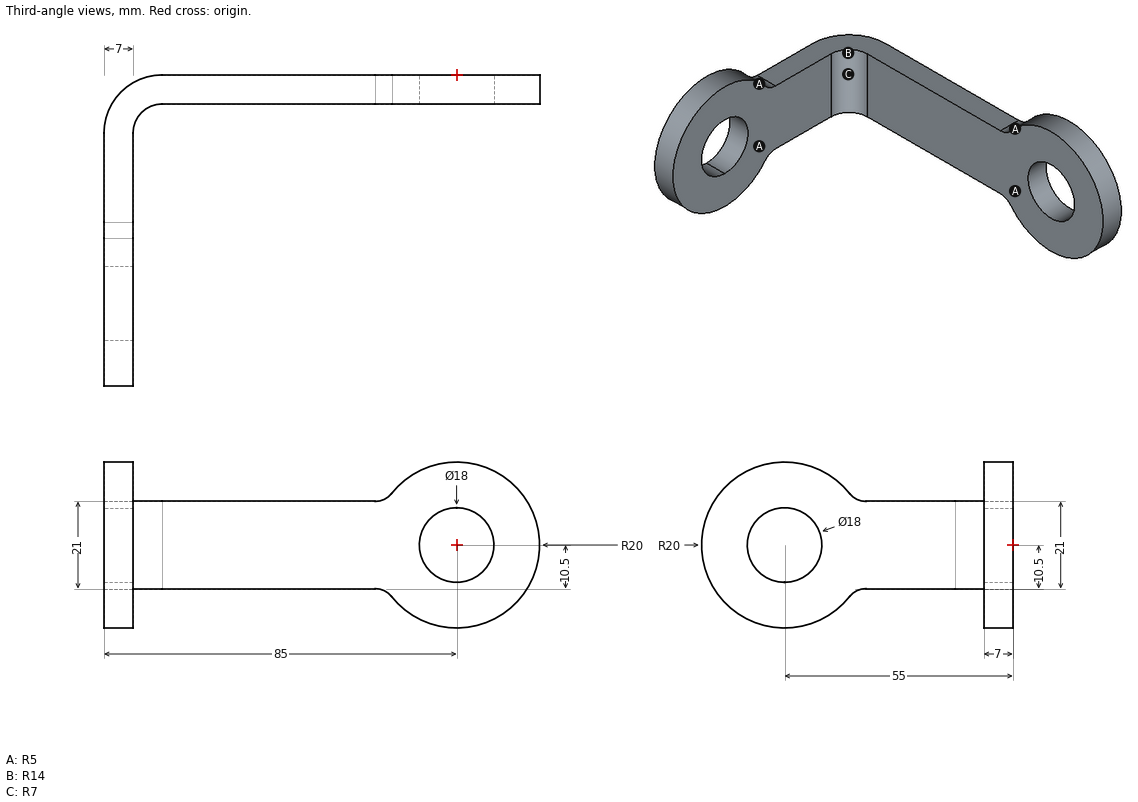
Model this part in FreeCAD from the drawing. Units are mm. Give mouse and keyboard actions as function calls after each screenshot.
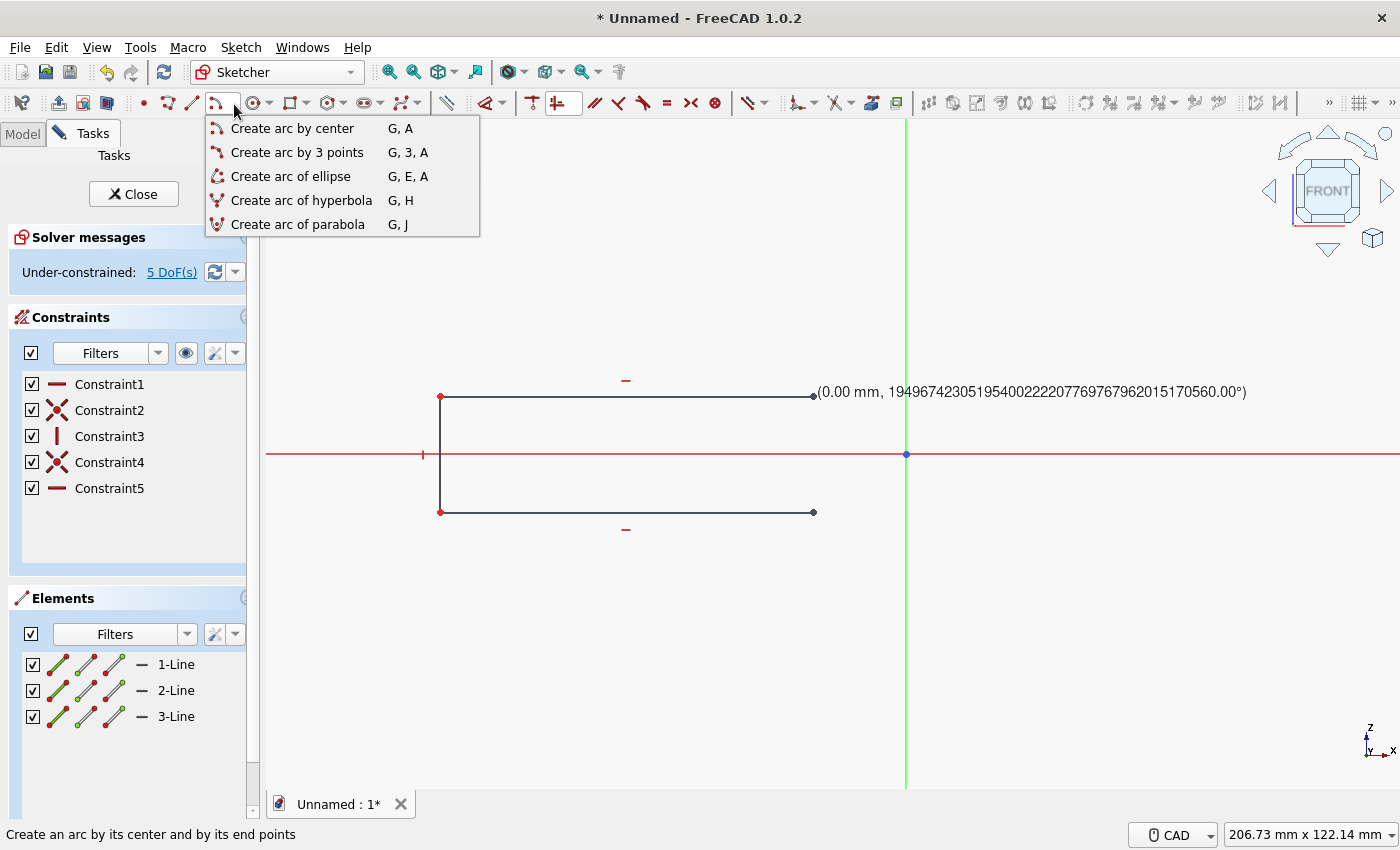
click(342, 152)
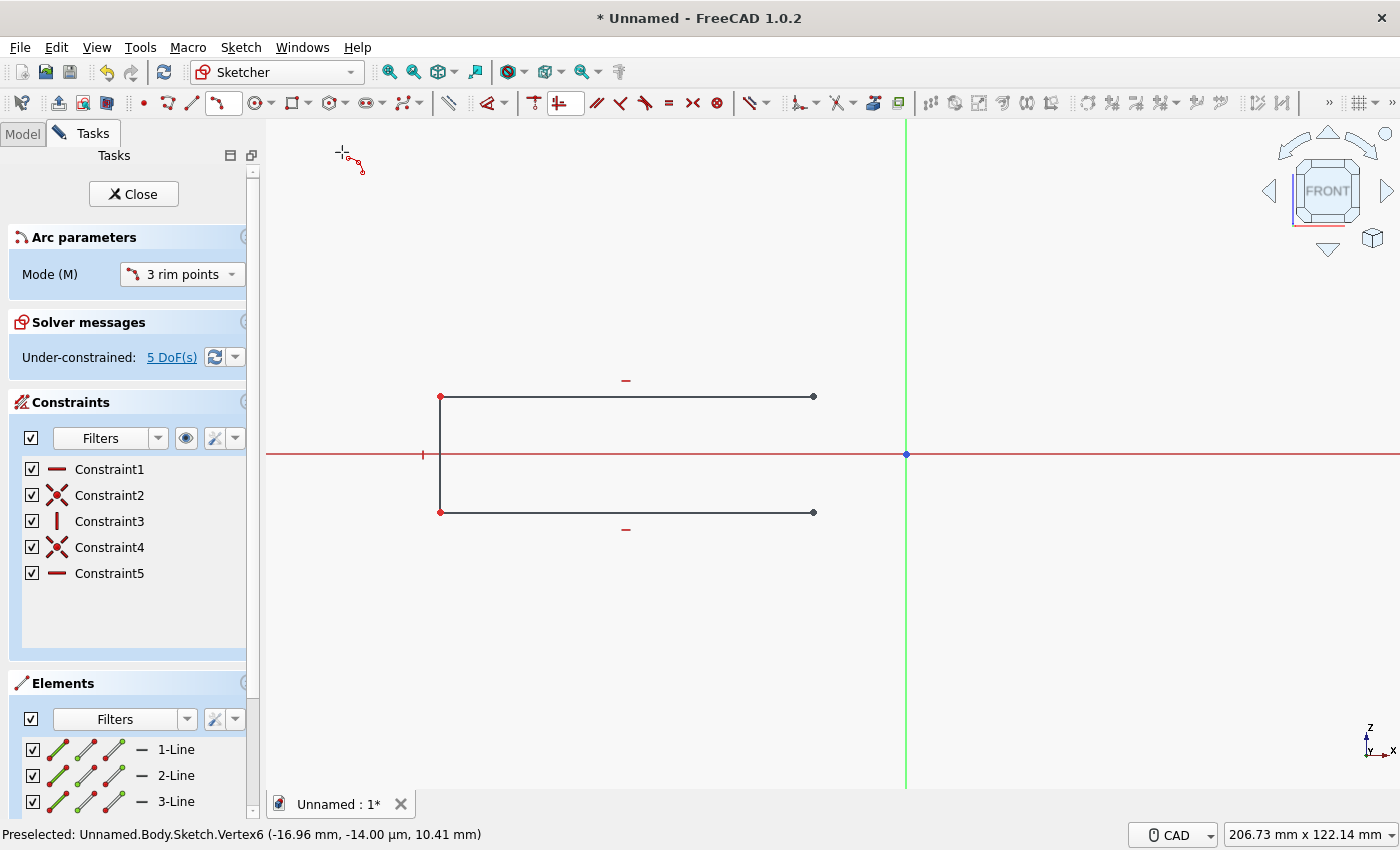
click(813, 397)
click(813, 513)
click(1001, 508)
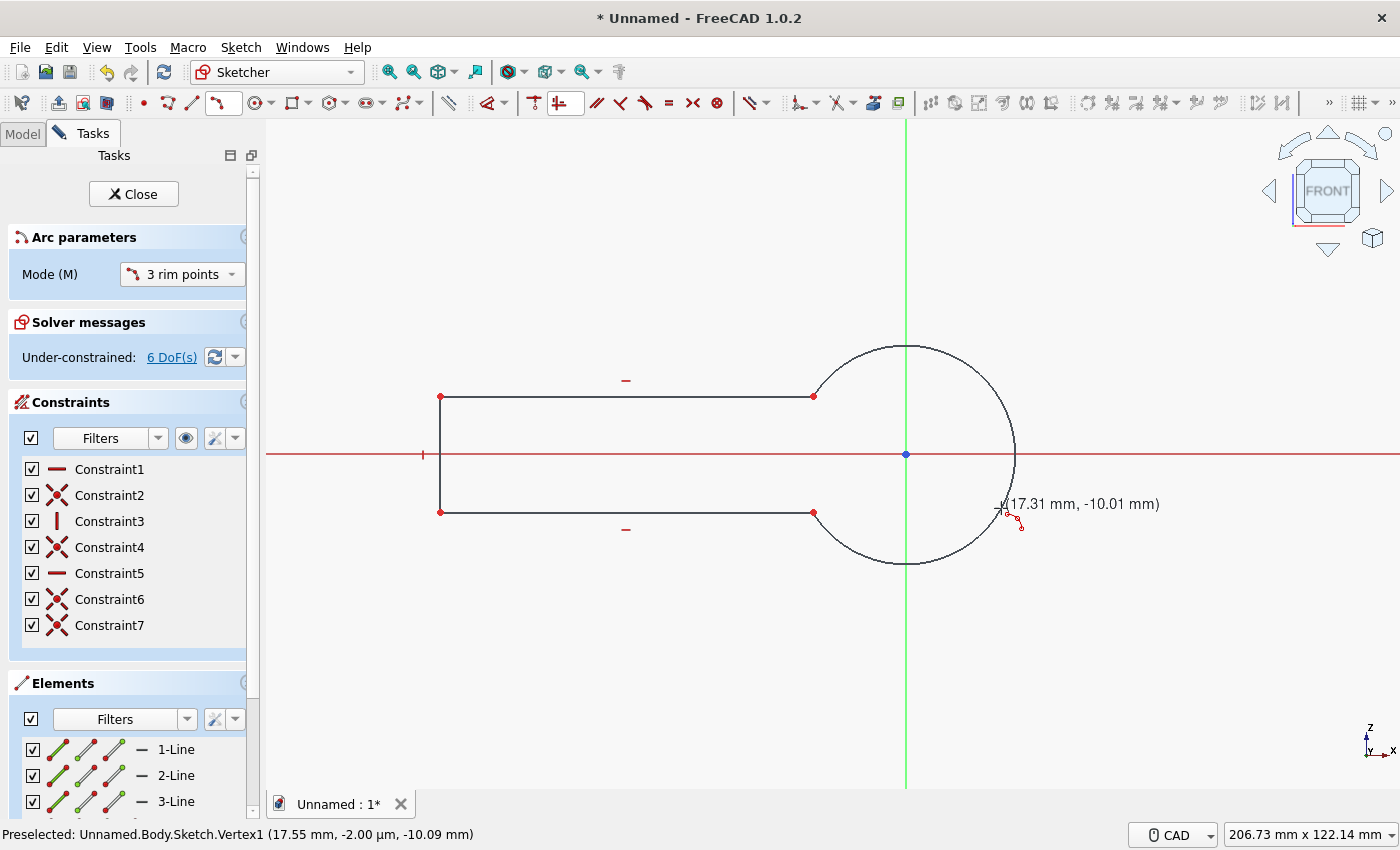
click(256, 104)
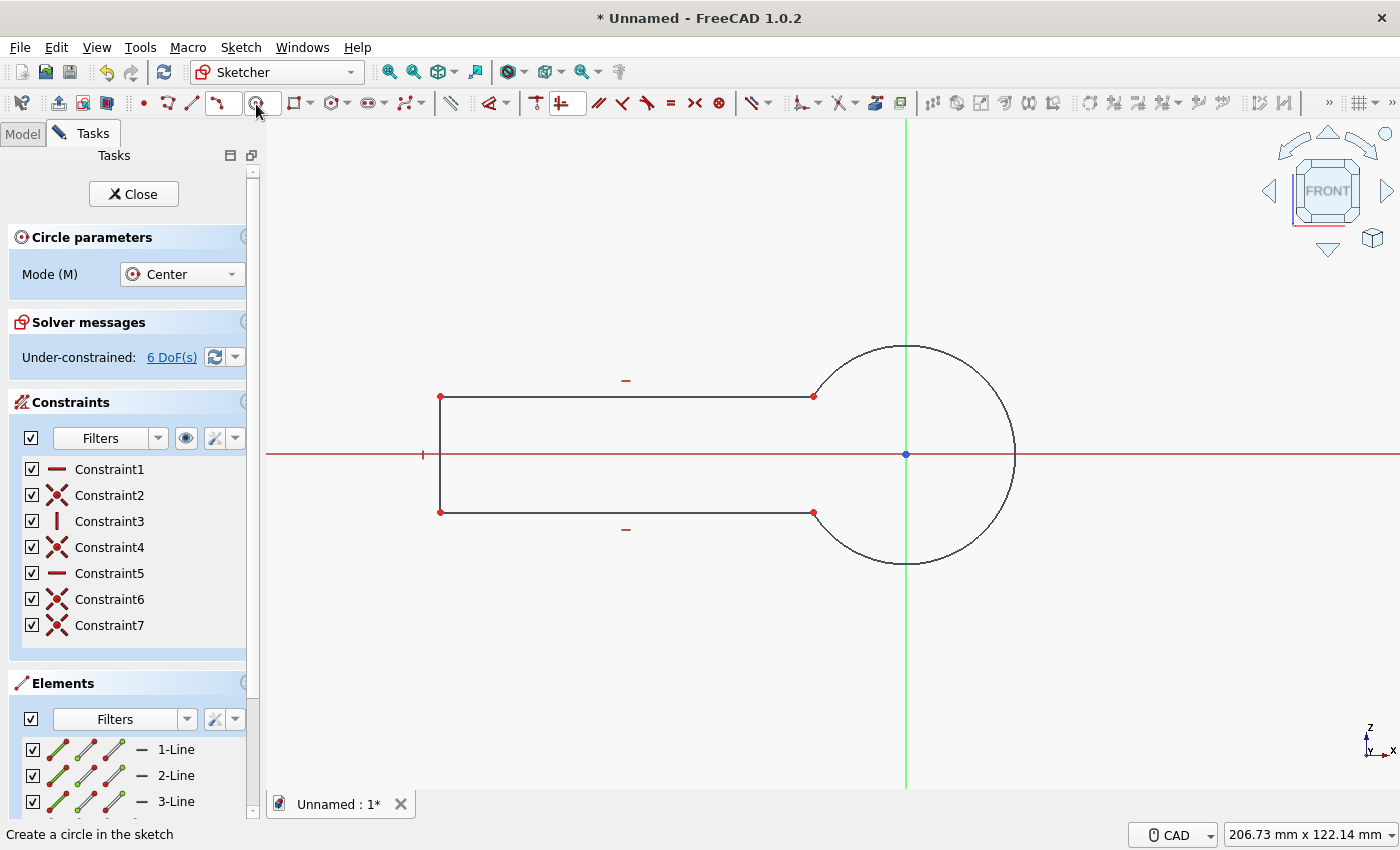
click(906, 454)
move(941, 419)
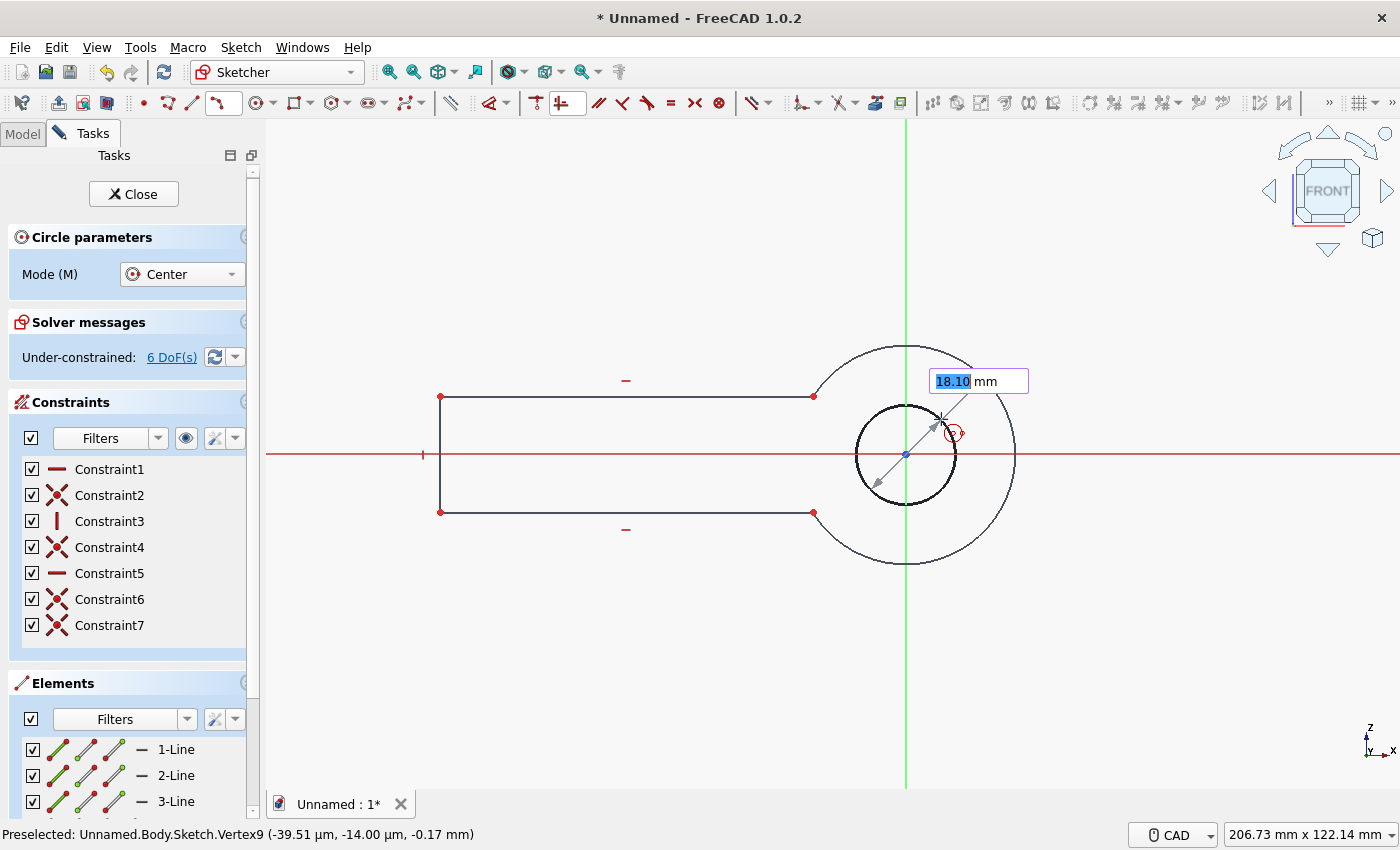
text(18)
key(Return)
key(Escape)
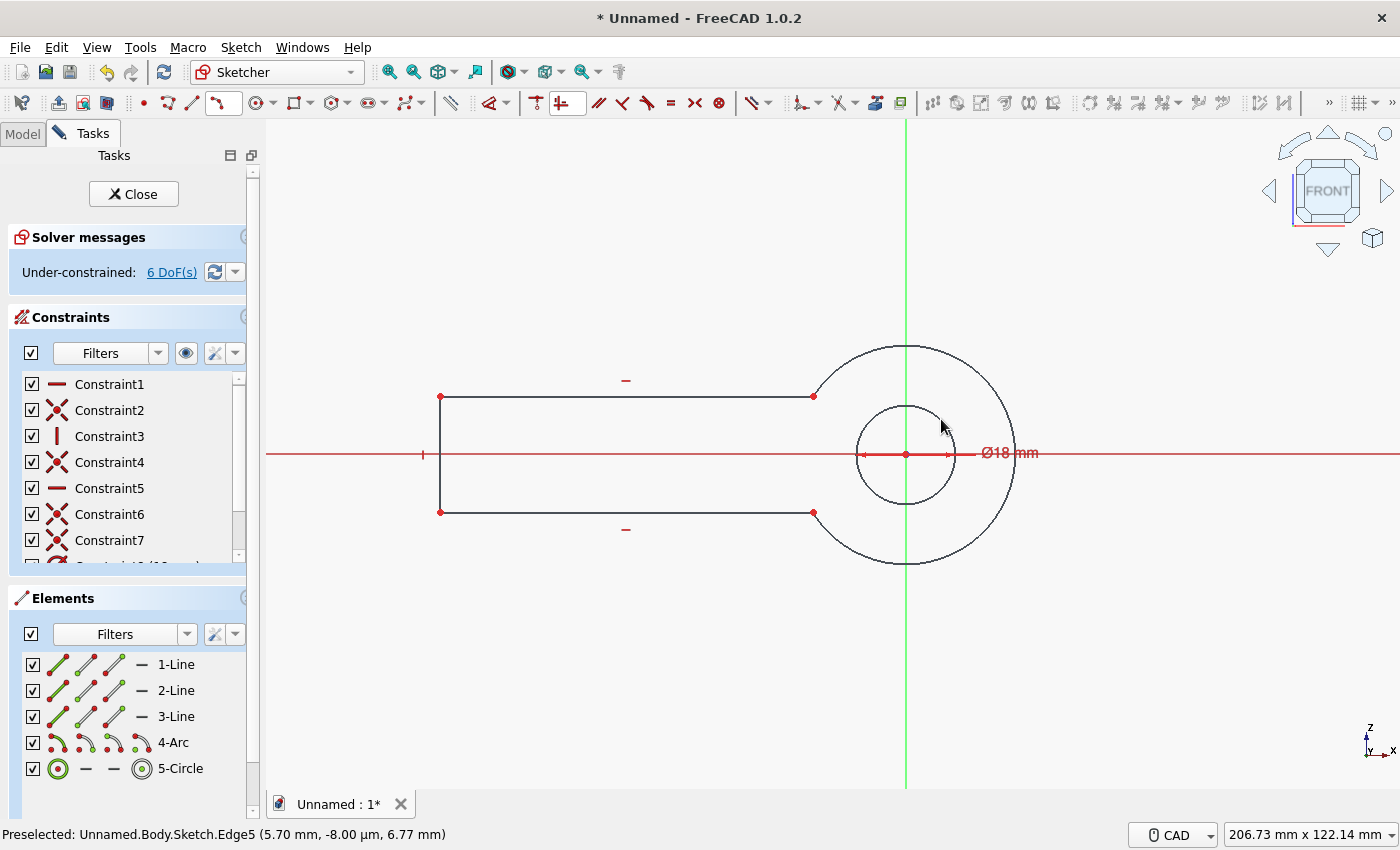
drag(896, 444, 916, 465)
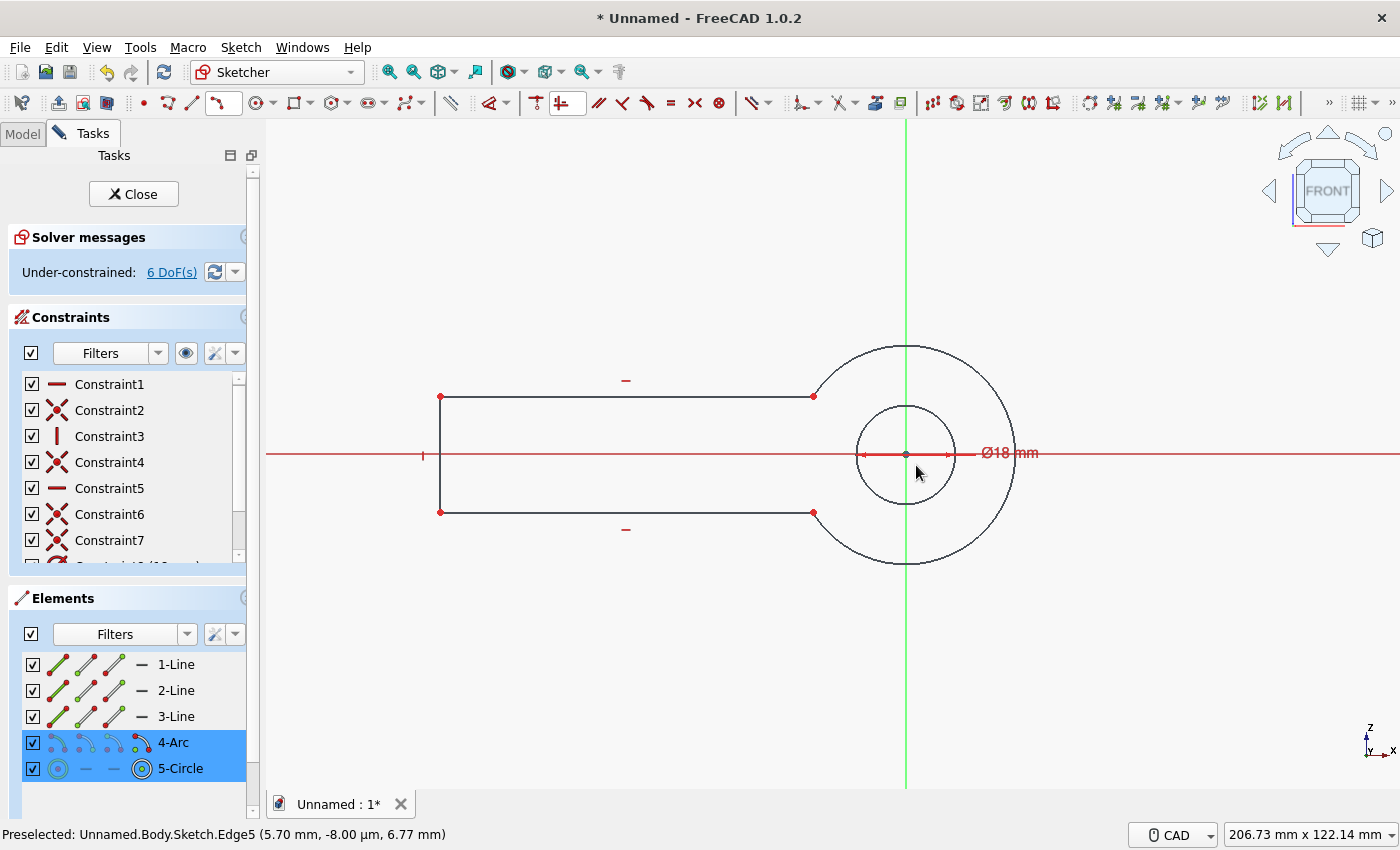
click(536, 104)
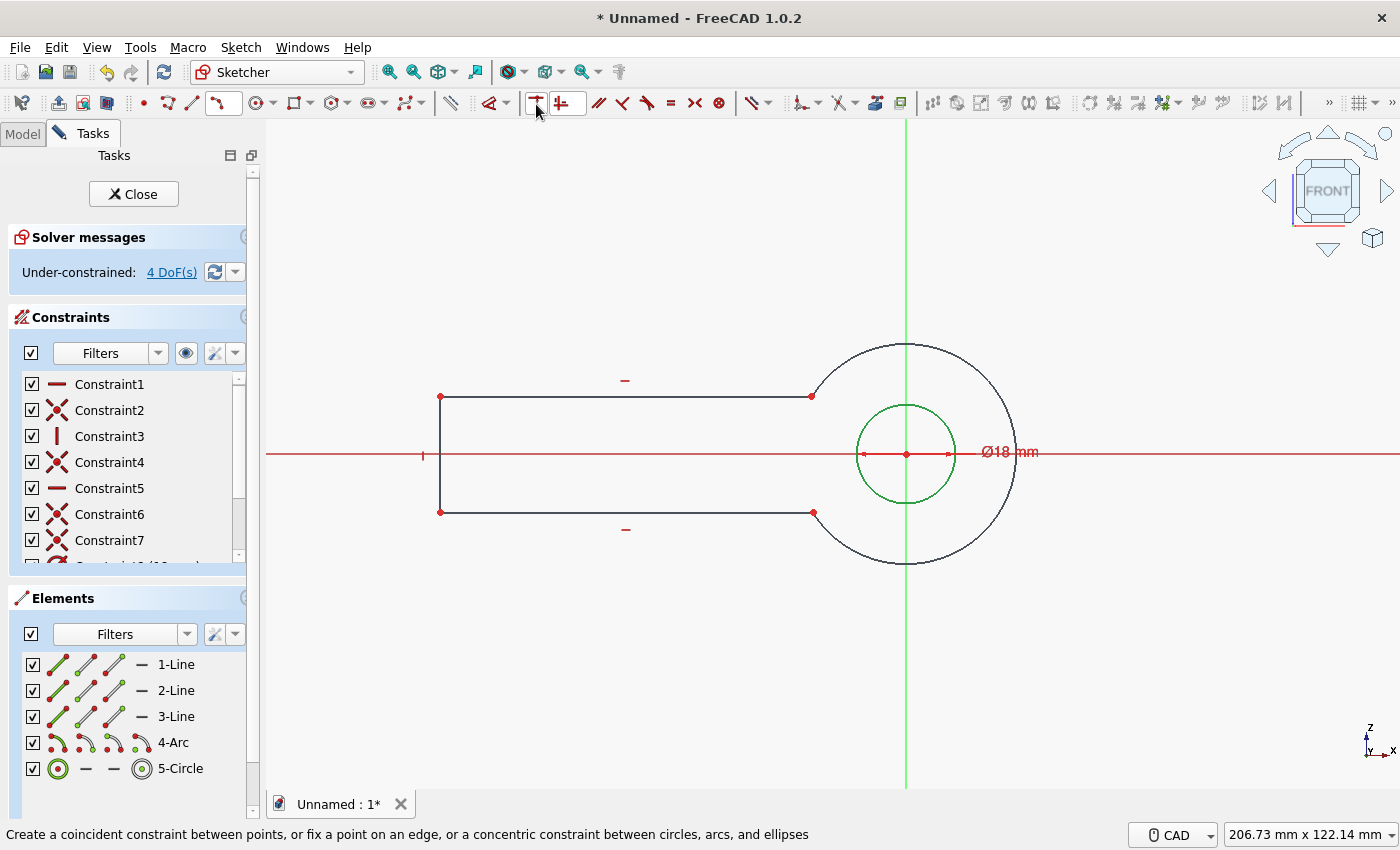
click(490, 104)